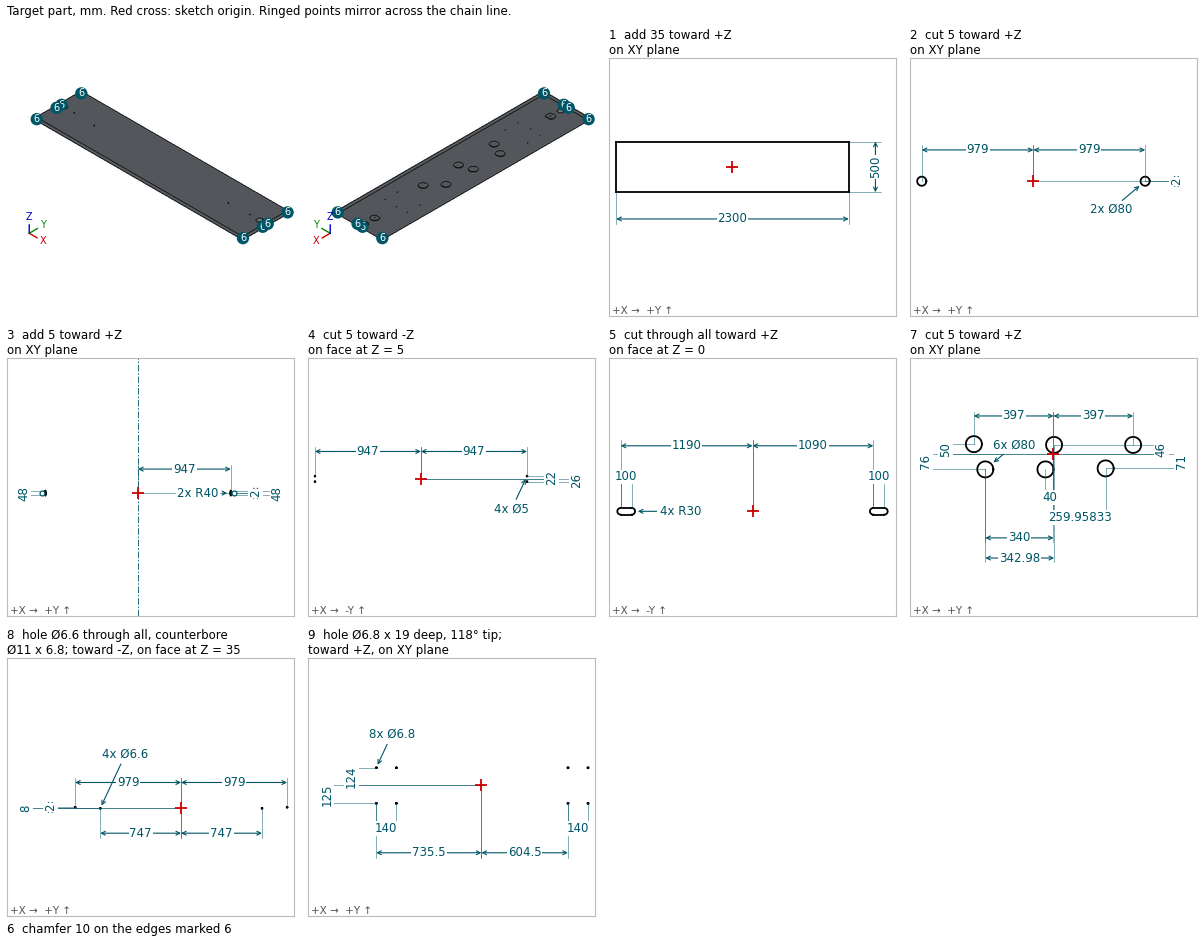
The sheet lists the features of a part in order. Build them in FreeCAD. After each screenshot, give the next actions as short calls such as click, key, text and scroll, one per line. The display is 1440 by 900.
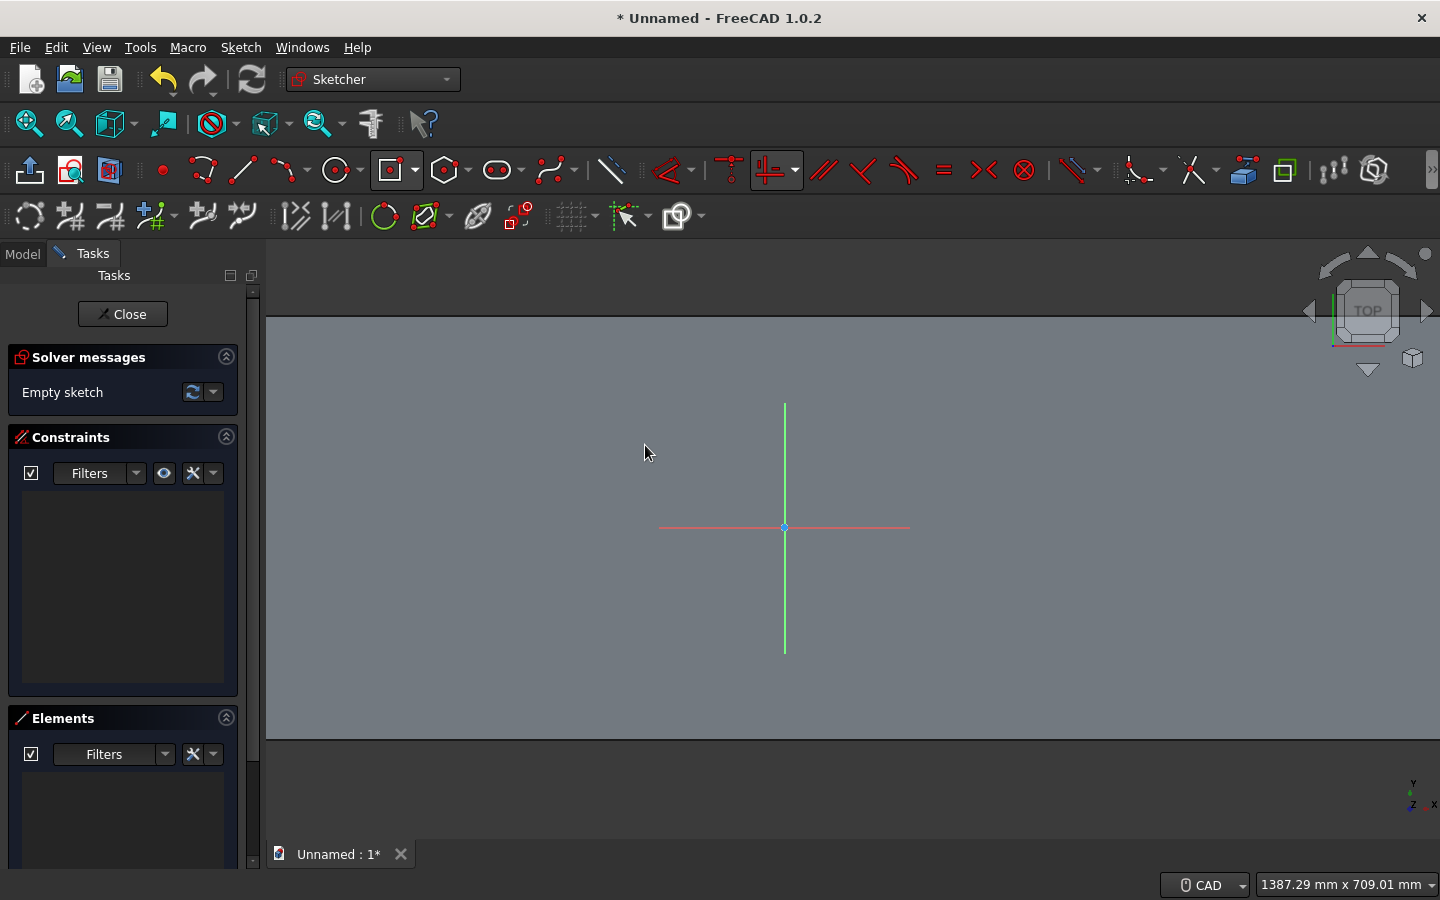
key(g)
key(c)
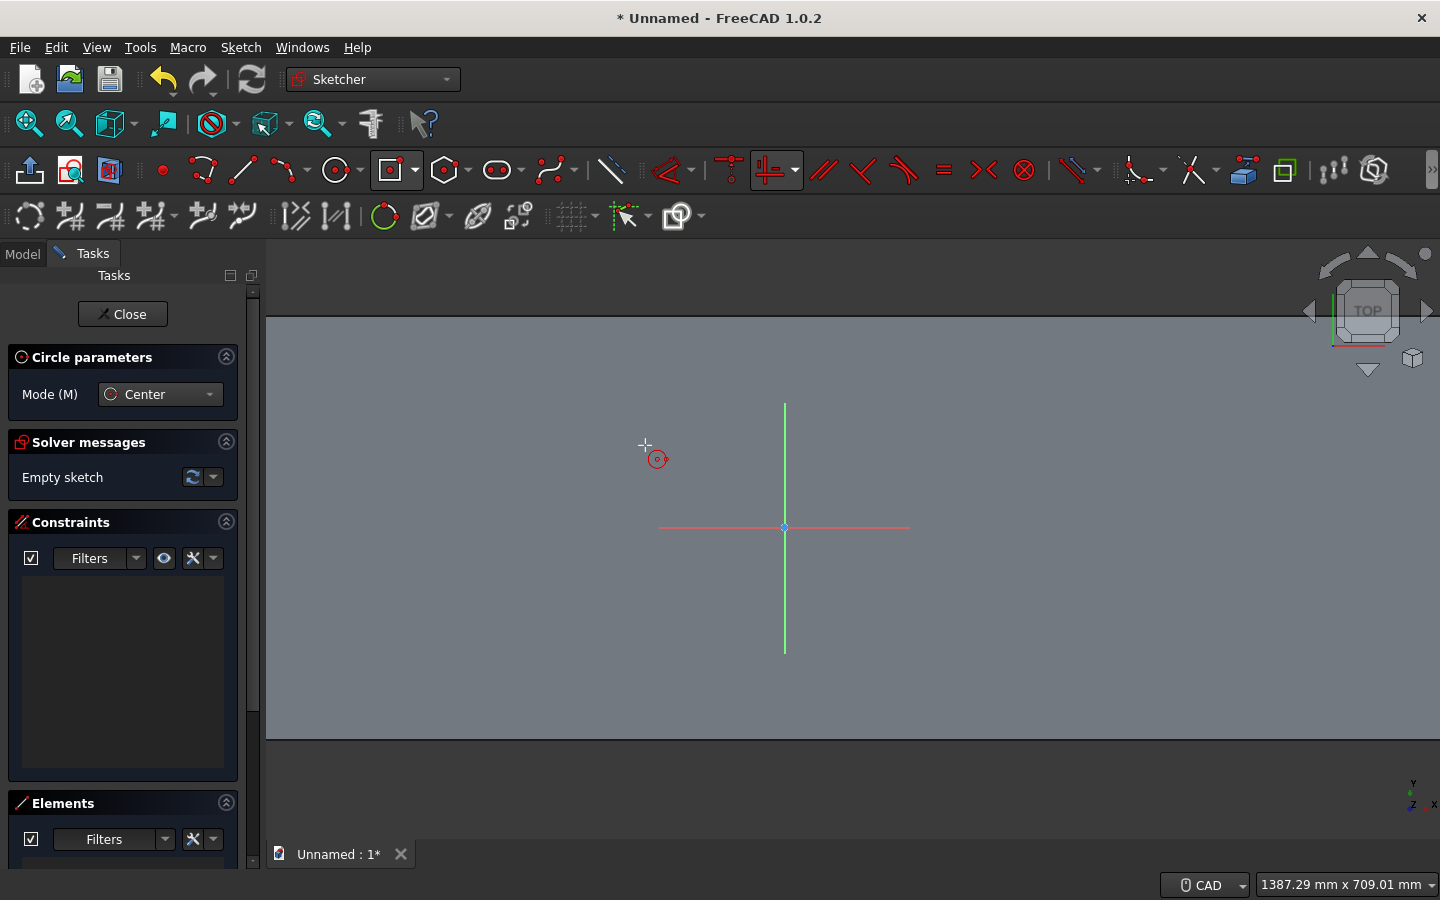
click(497, 592)
click(521, 568)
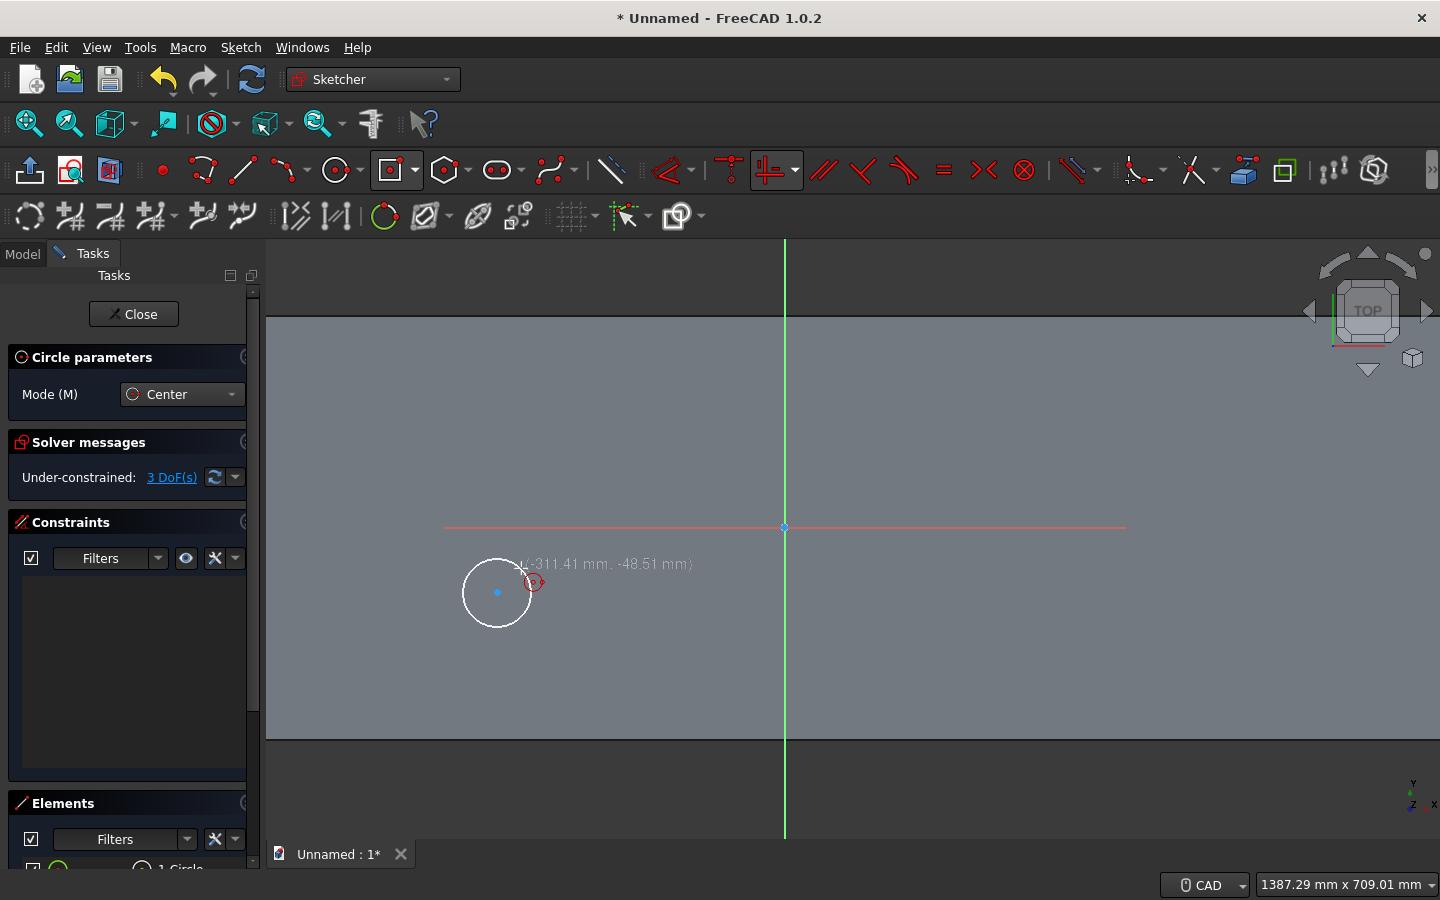
click(449, 486)
click(473, 462)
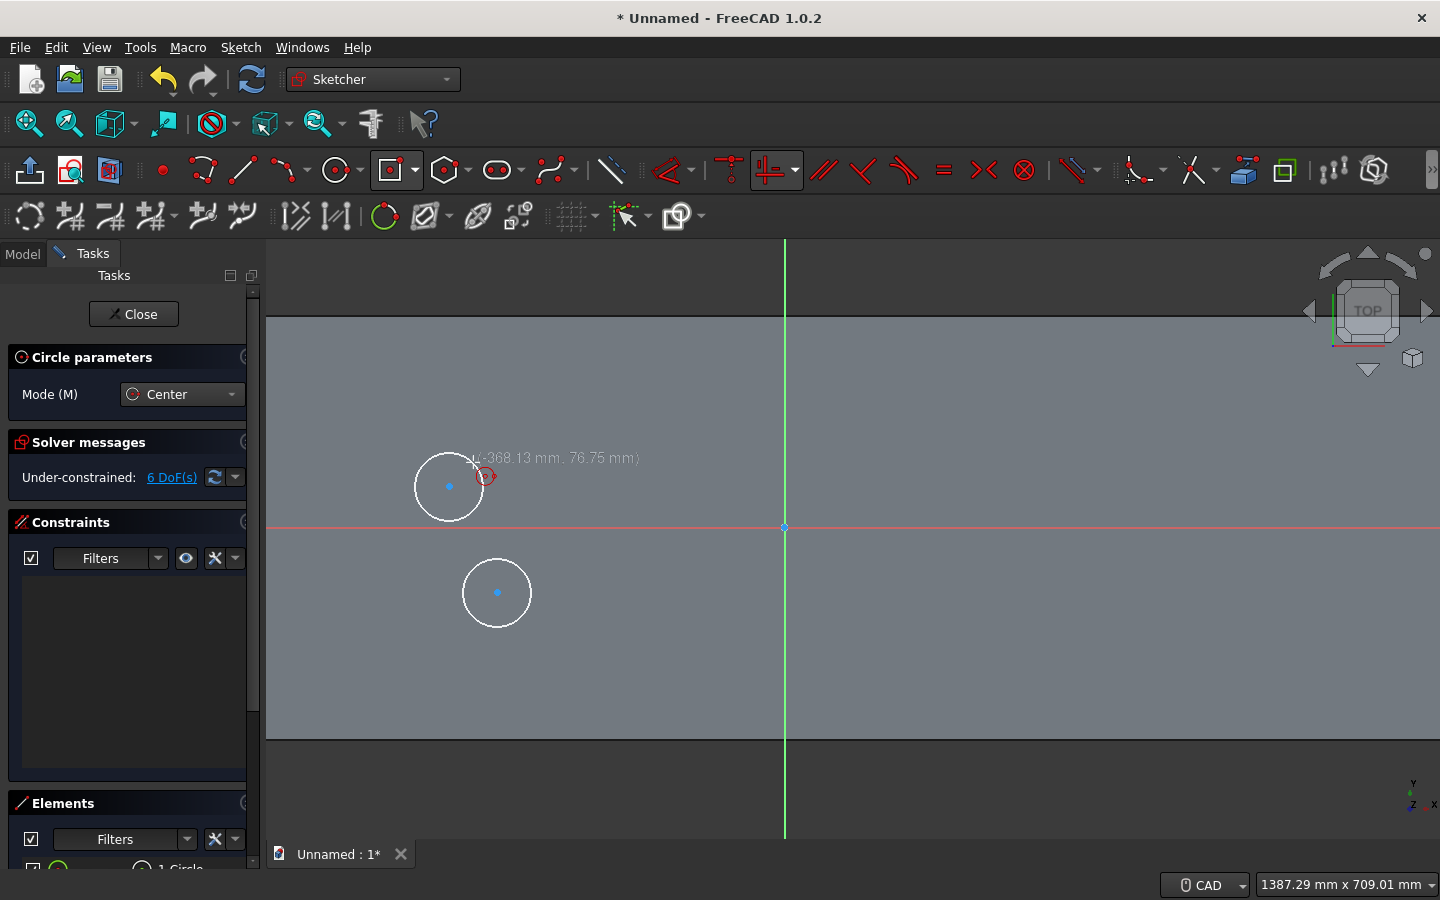
scroll(787, 489, up, 10)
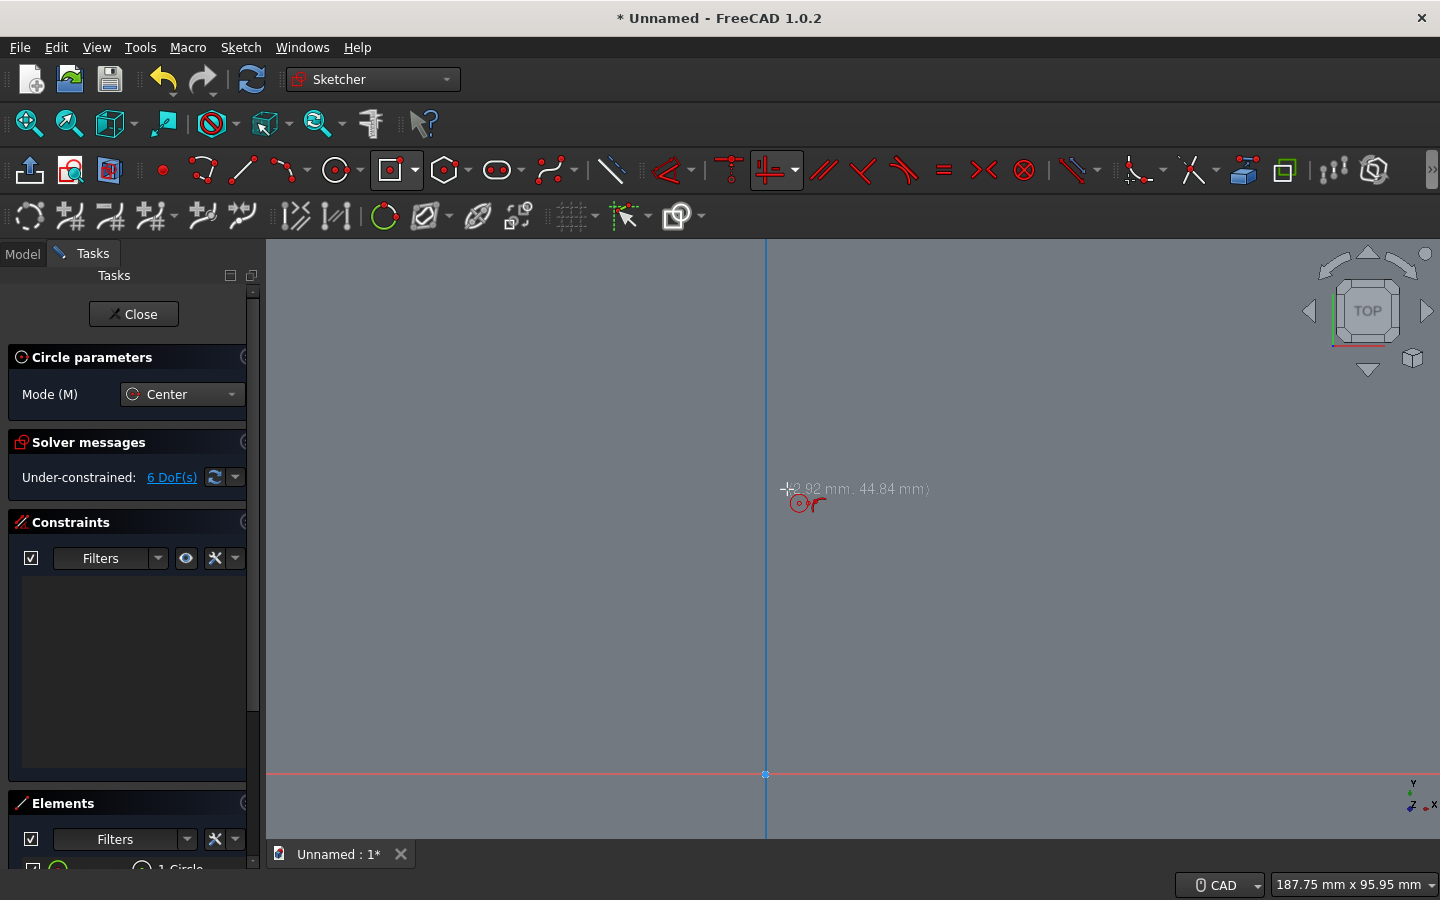
click(785, 486)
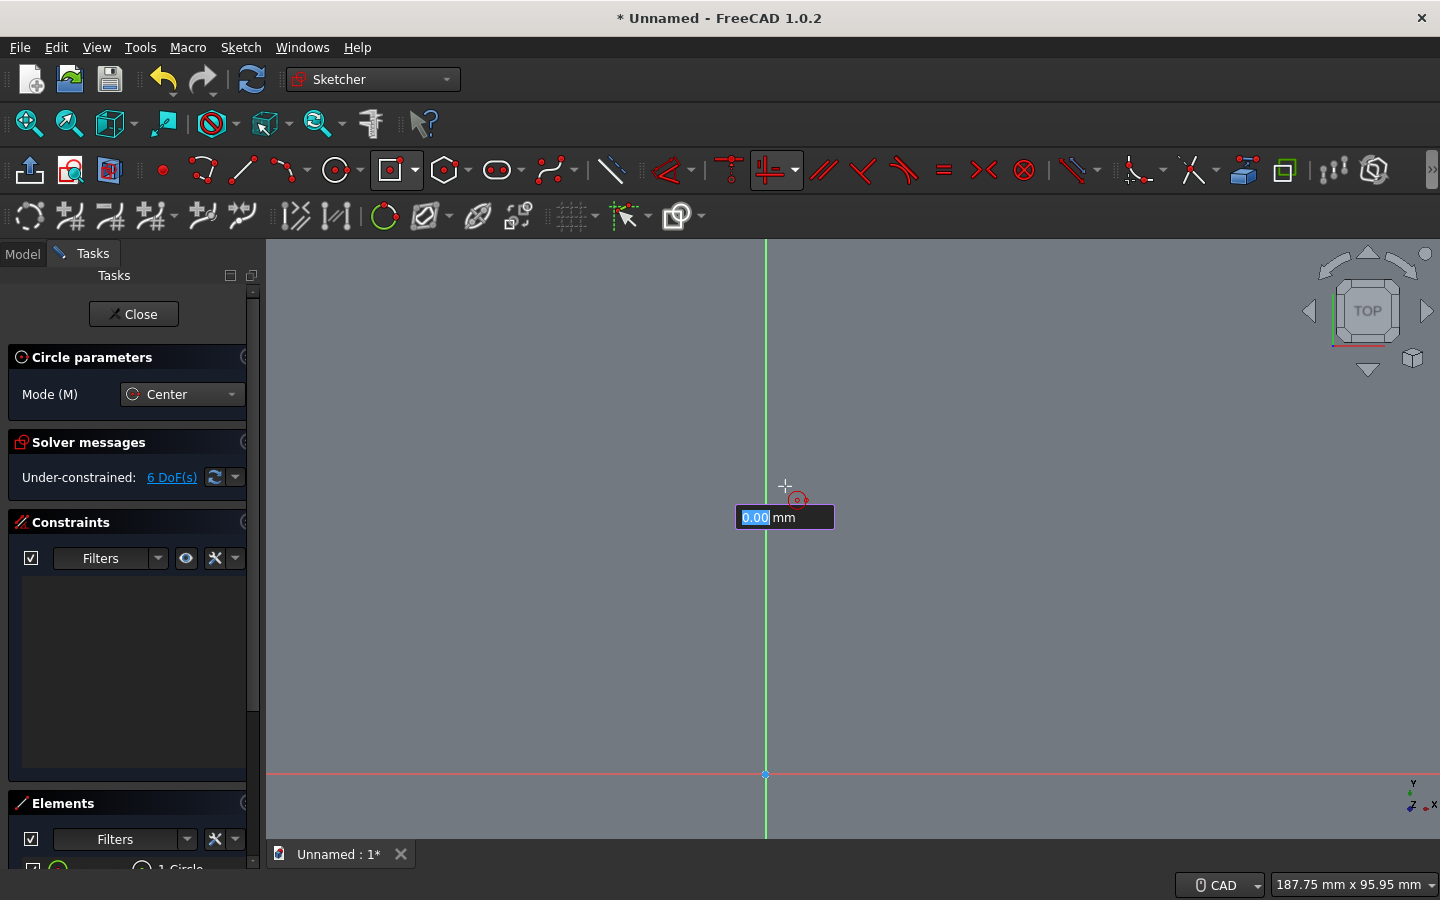
scroll(787, 489, down, 10)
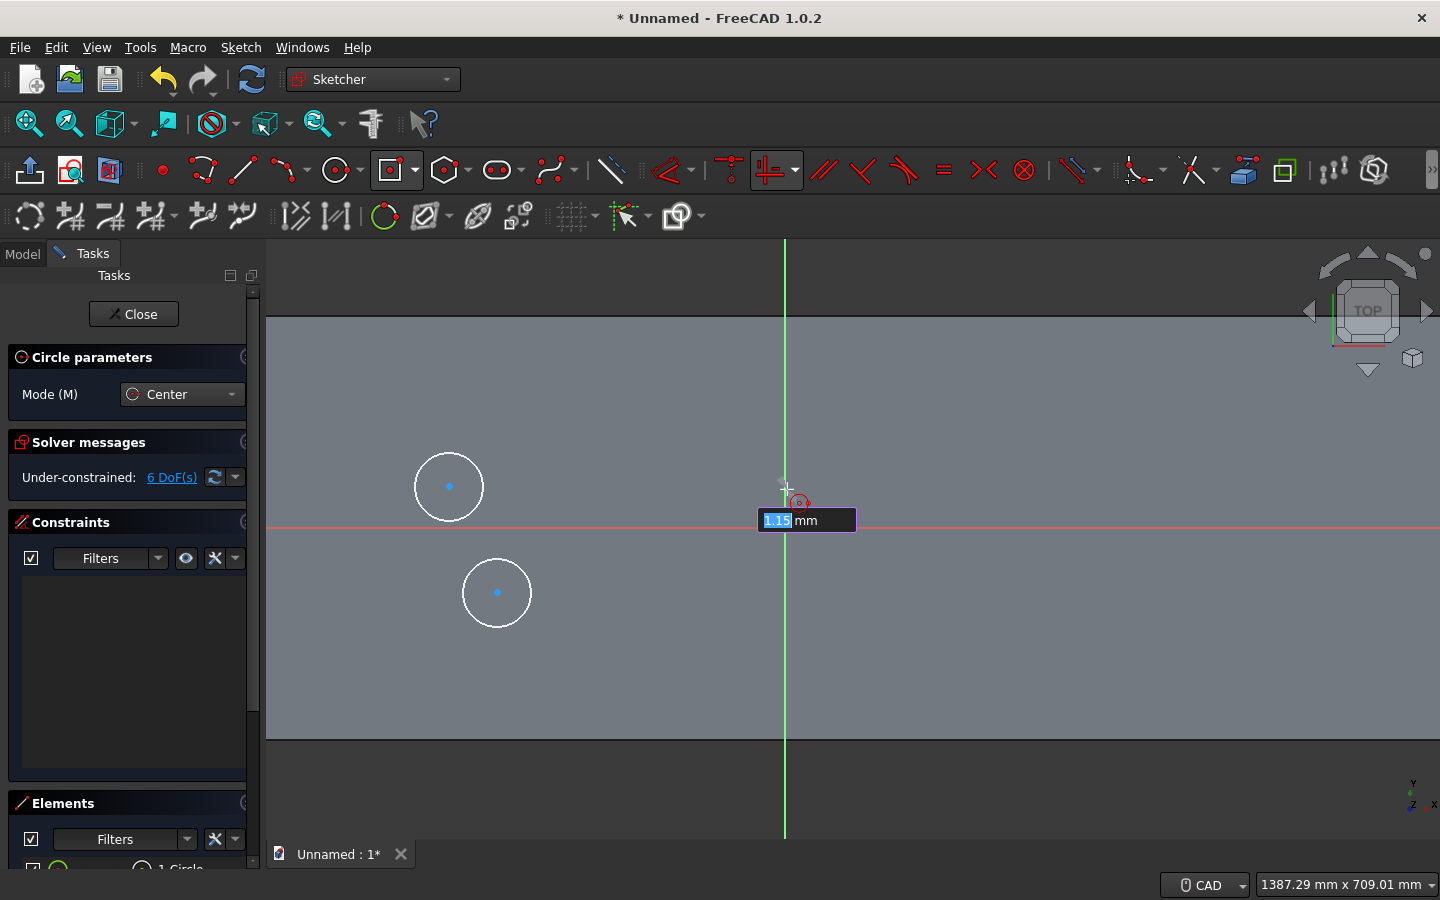
click(811, 465)